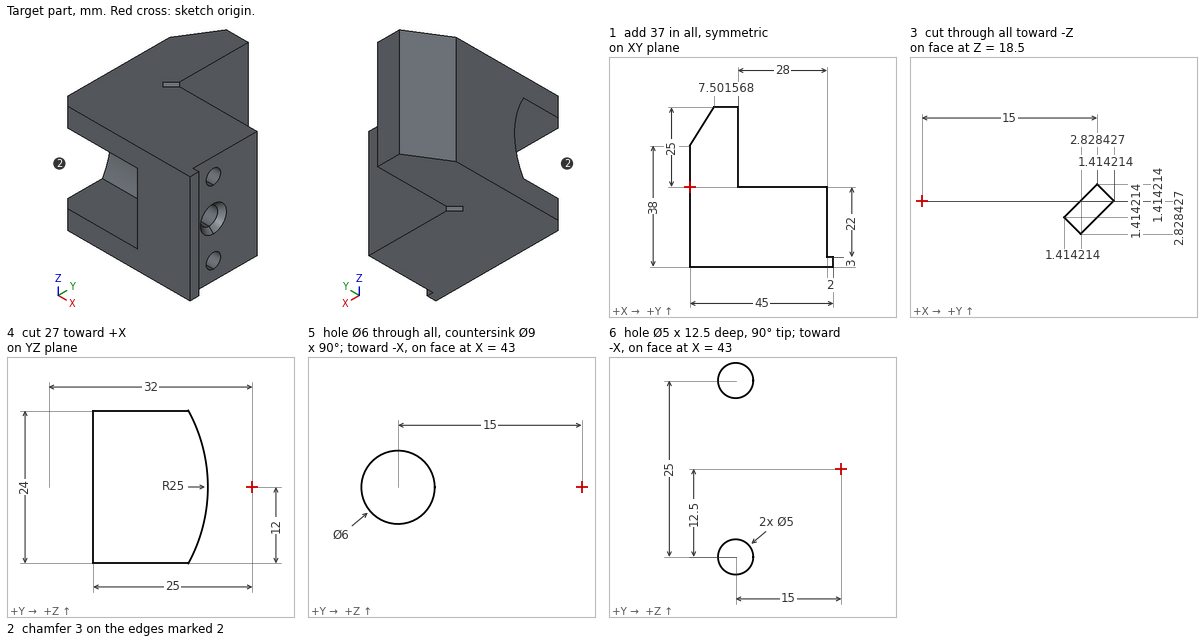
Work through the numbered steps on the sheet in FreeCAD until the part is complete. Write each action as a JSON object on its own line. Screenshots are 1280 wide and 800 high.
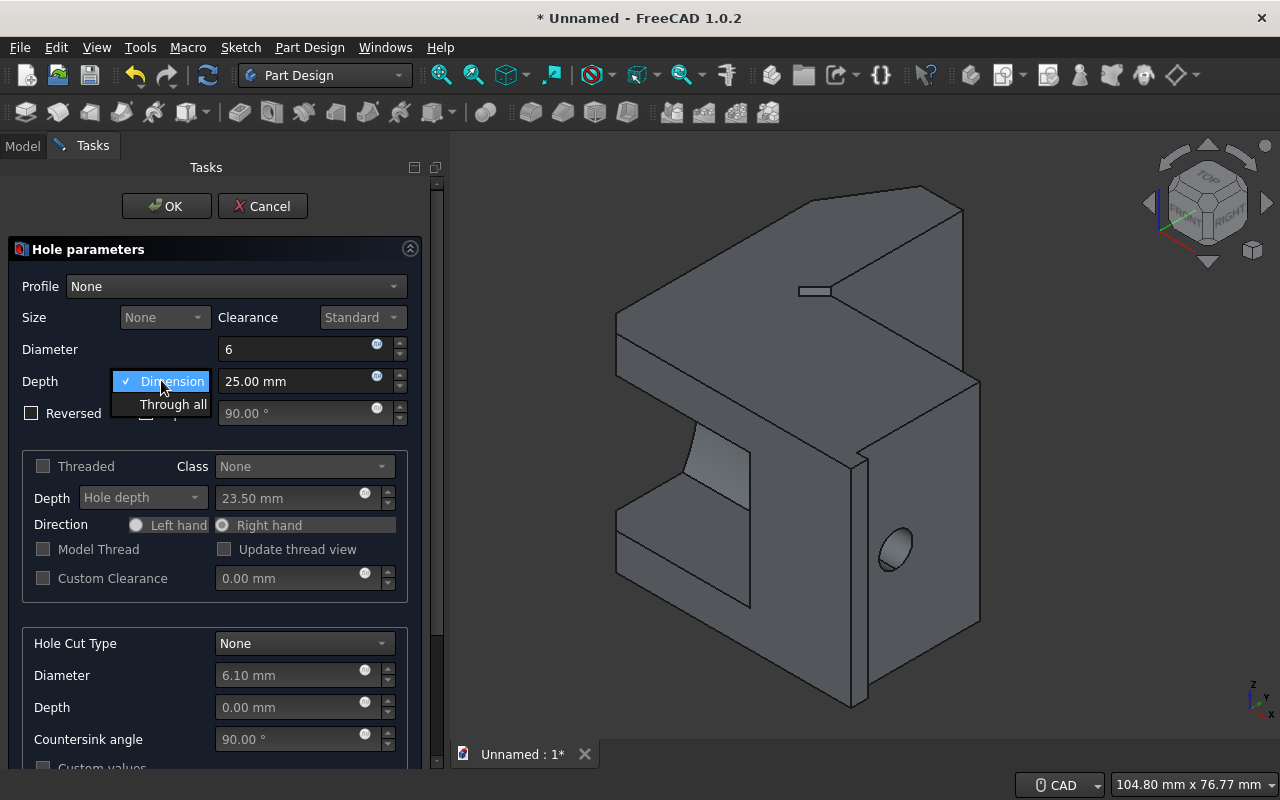
{"action": "left_click", "coordinate": [160, 404]}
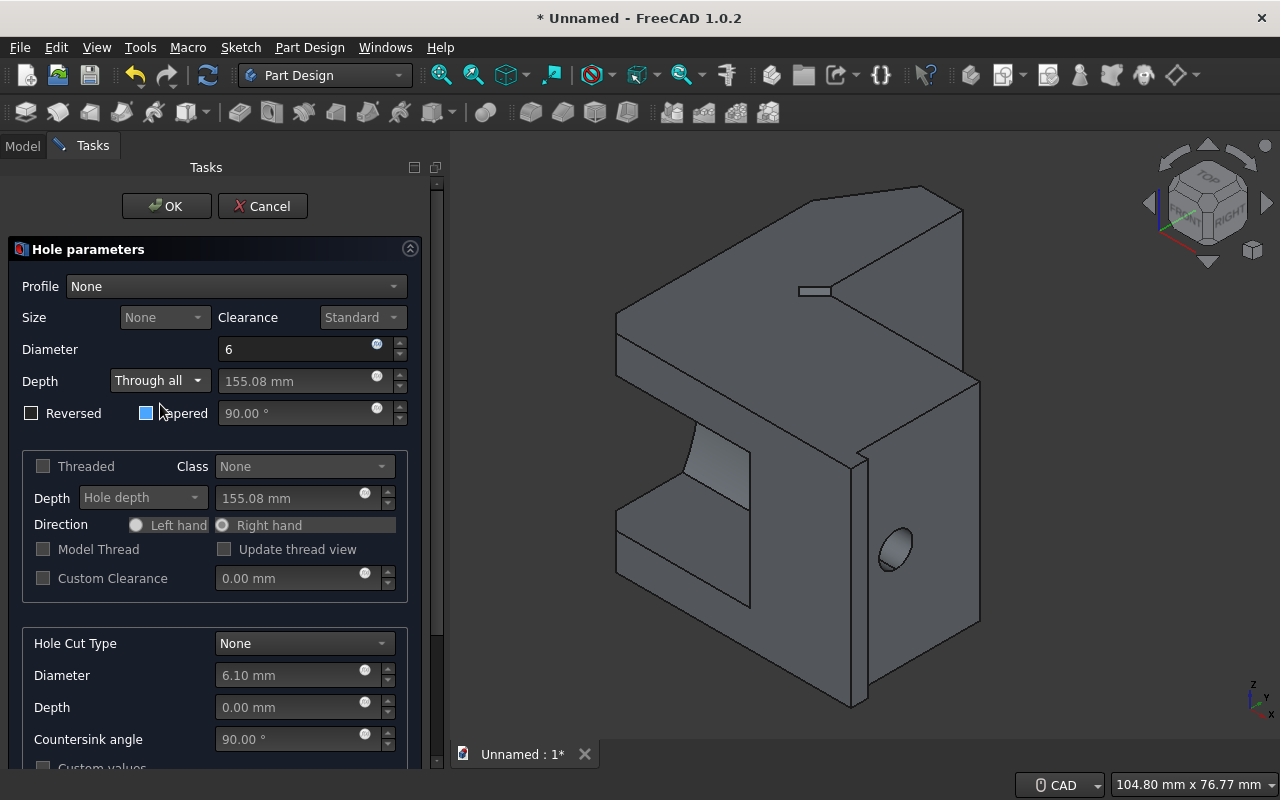
{"action": "left_click", "coordinate": [306, 644]}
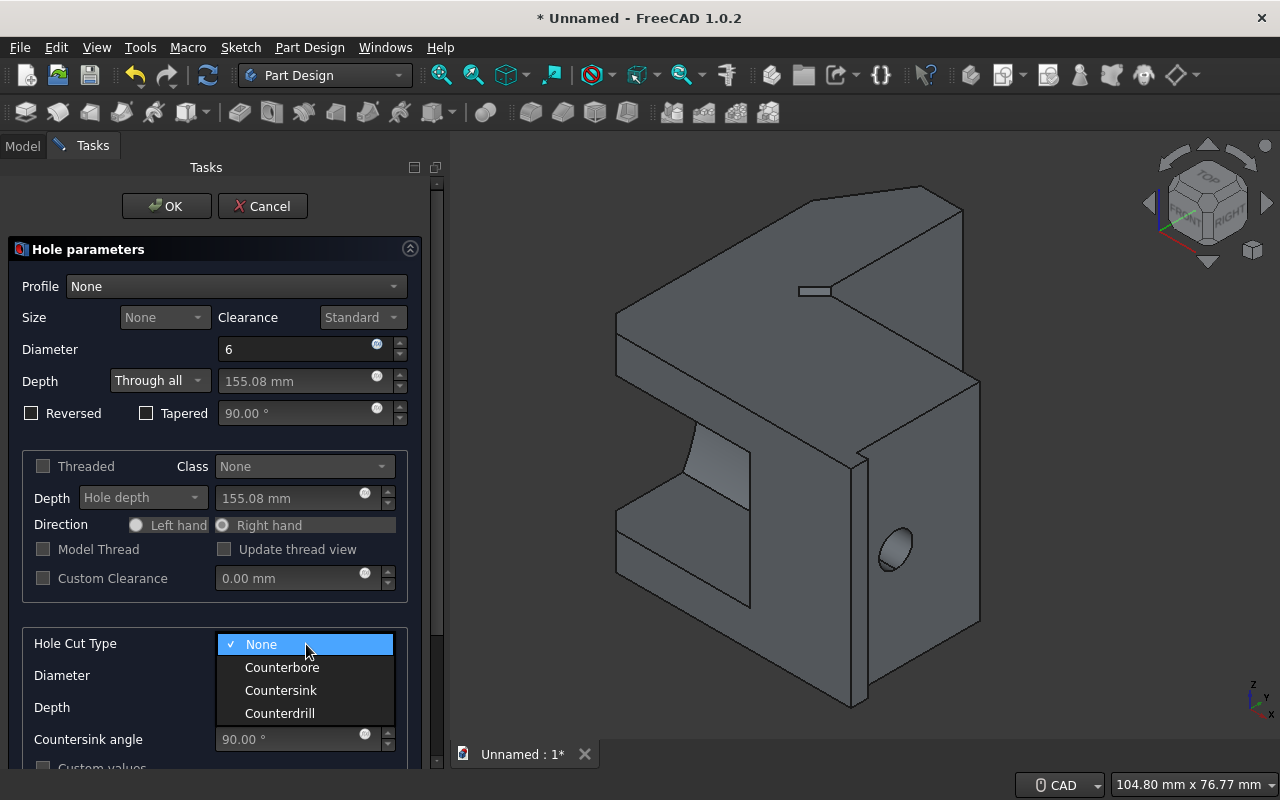
{"action": "left_click", "coordinate": [304, 690]}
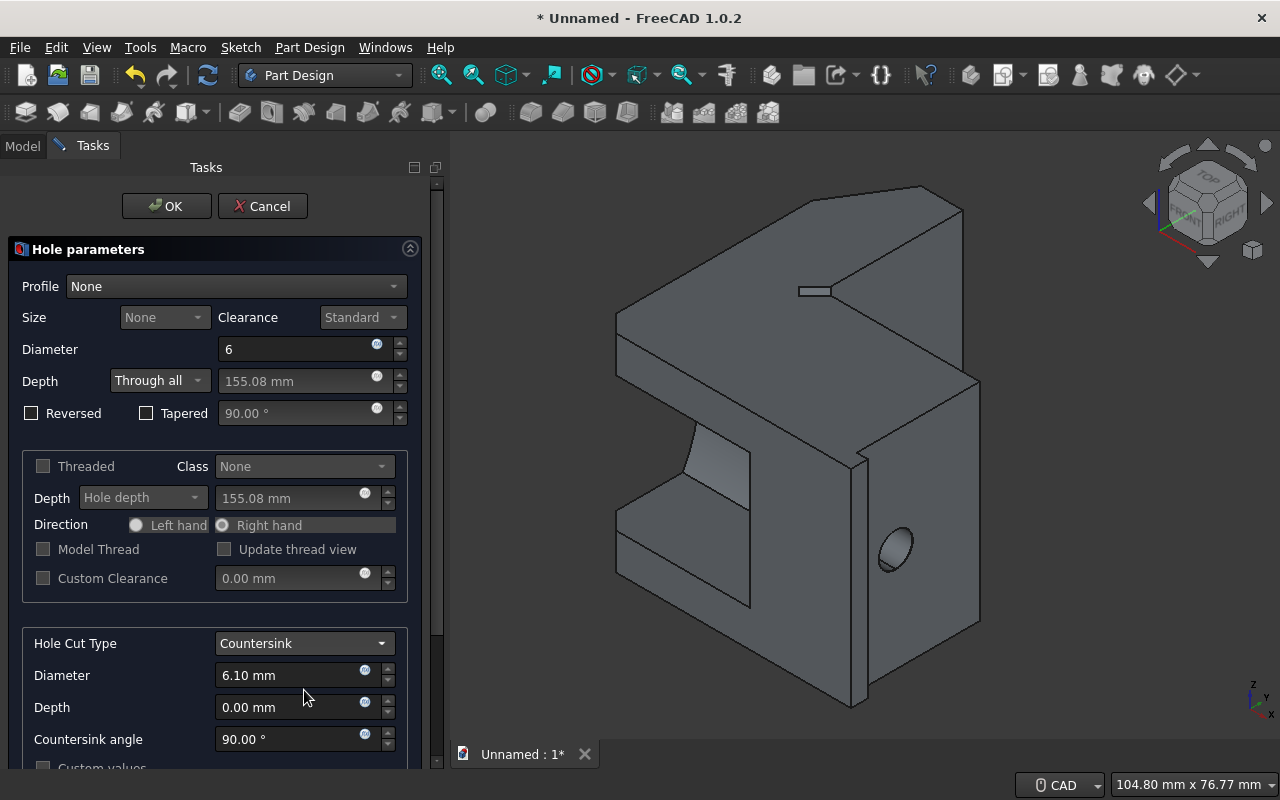
{"action": "triple_click", "coordinate": [298, 675]}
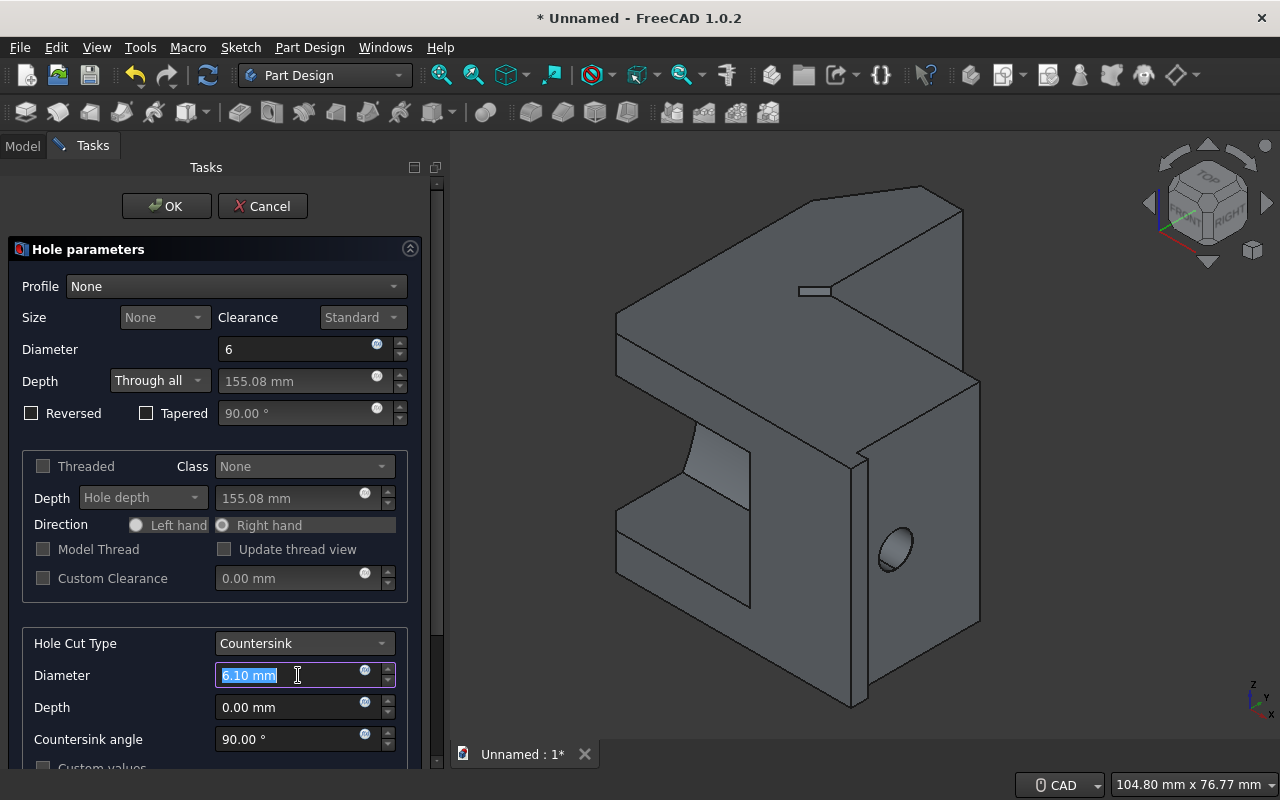
{"action": "type", "text": "9"}
{"action": "key", "text": "Tab"}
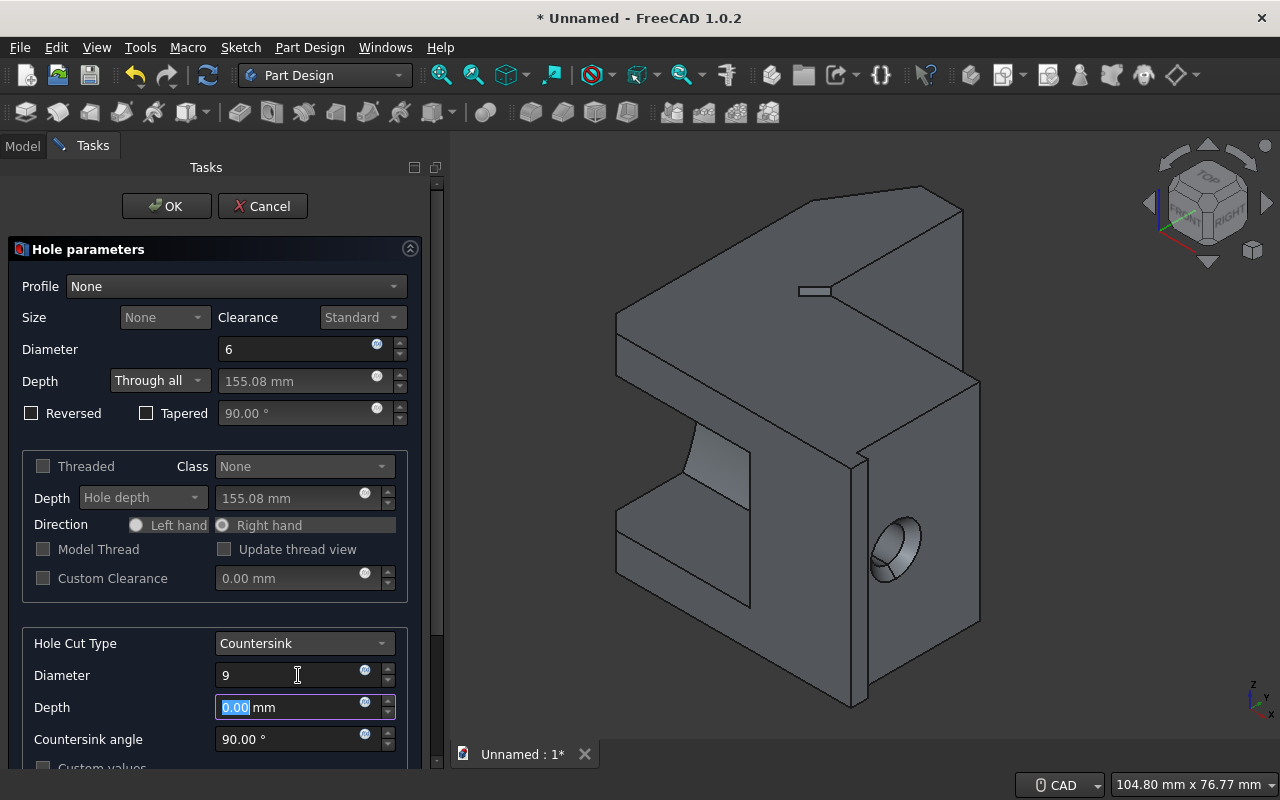
{"action": "left_click", "coordinate": [167, 206]}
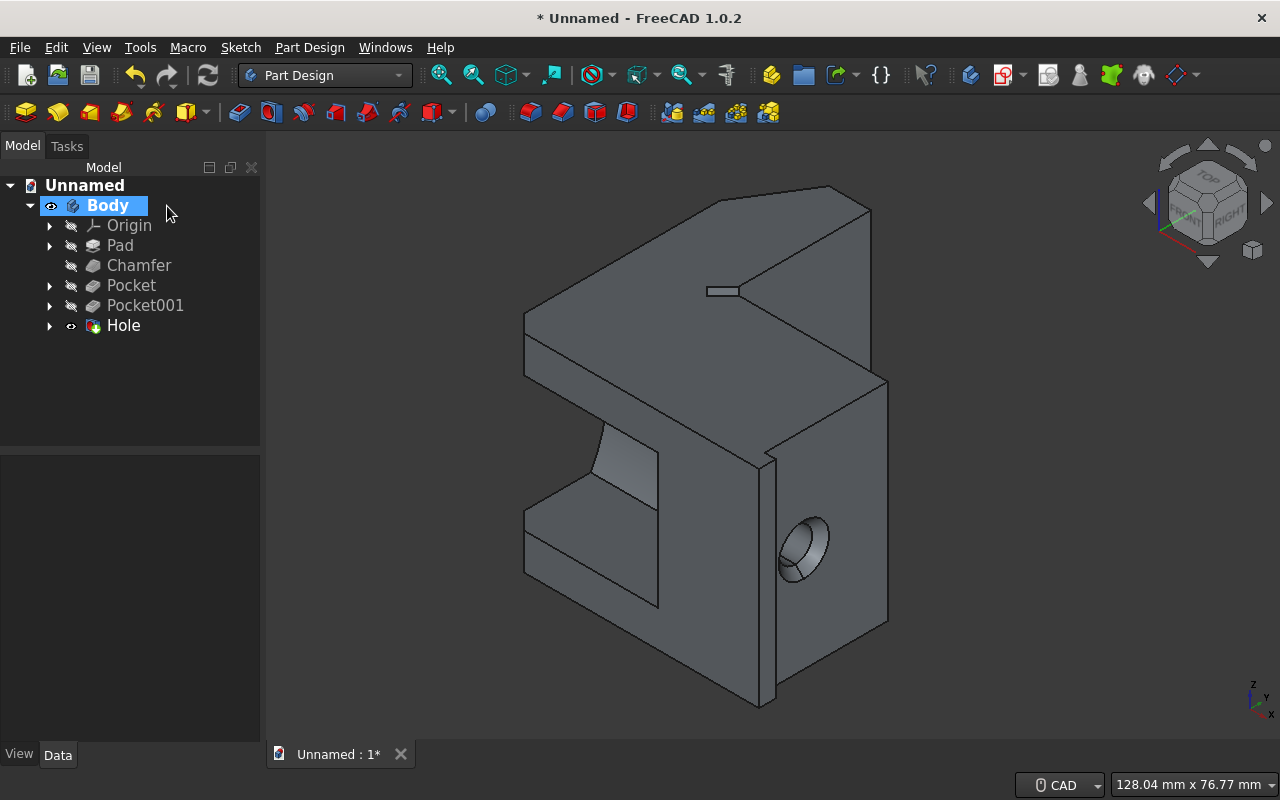
{"action": "left_click", "coordinate": [844, 457]}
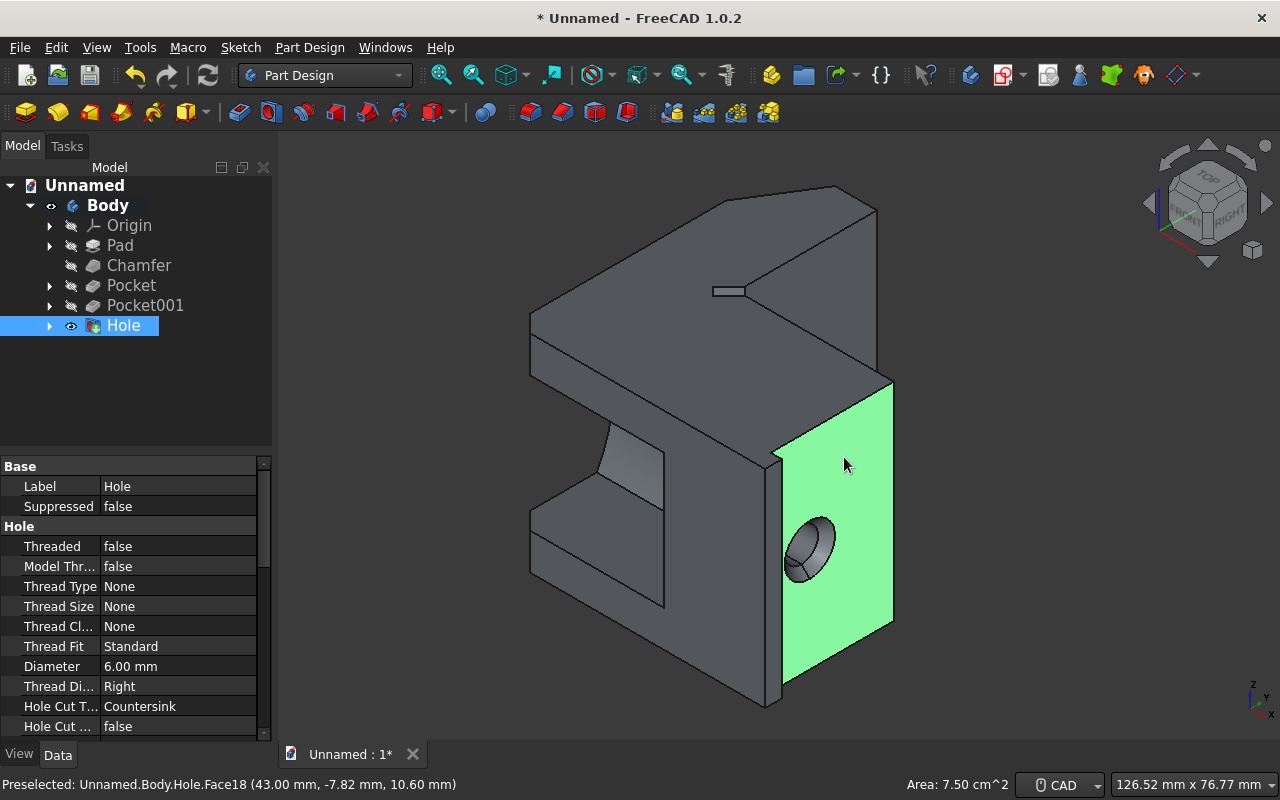
{"action": "left_click", "coordinate": [1004, 76]}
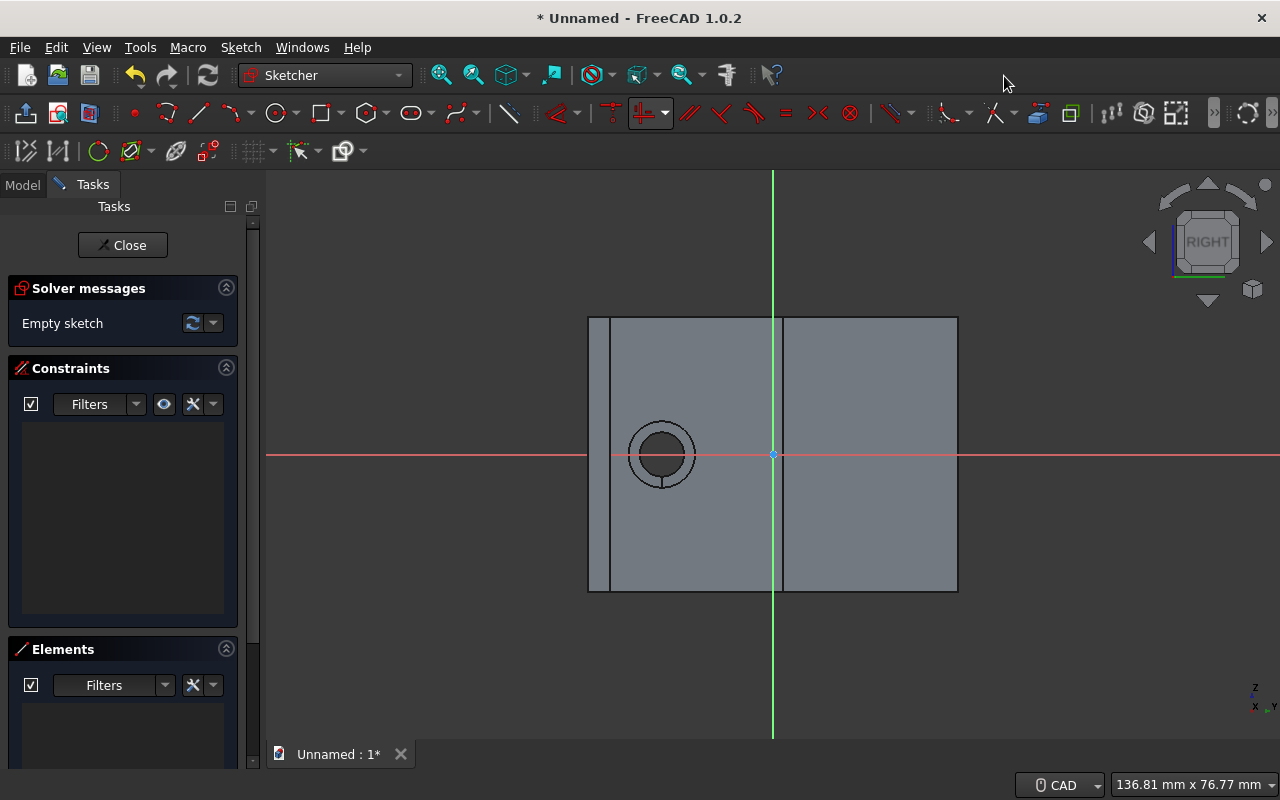
{"action": "scroll", "coordinate": [716, 454], "scroll_direction": "up", "scroll_amount": 2}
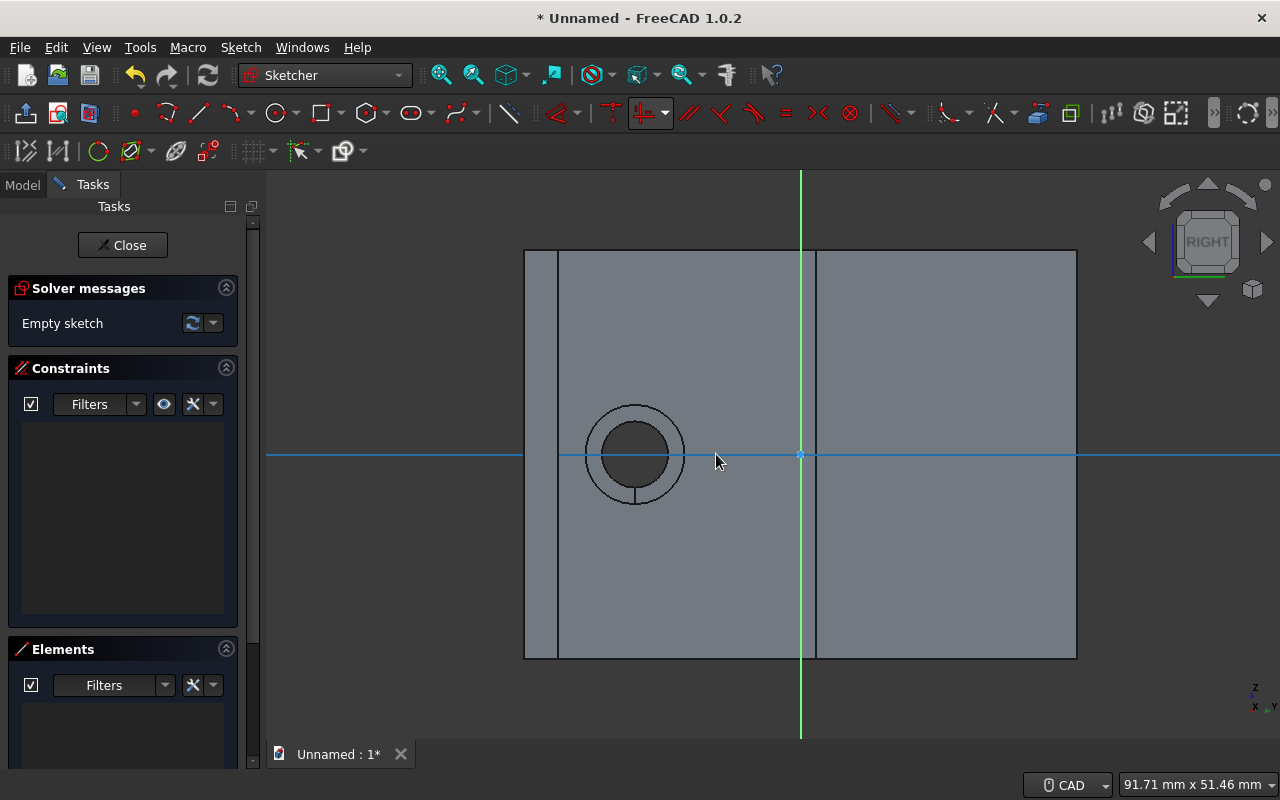
{"action": "key", "text": "g c"}